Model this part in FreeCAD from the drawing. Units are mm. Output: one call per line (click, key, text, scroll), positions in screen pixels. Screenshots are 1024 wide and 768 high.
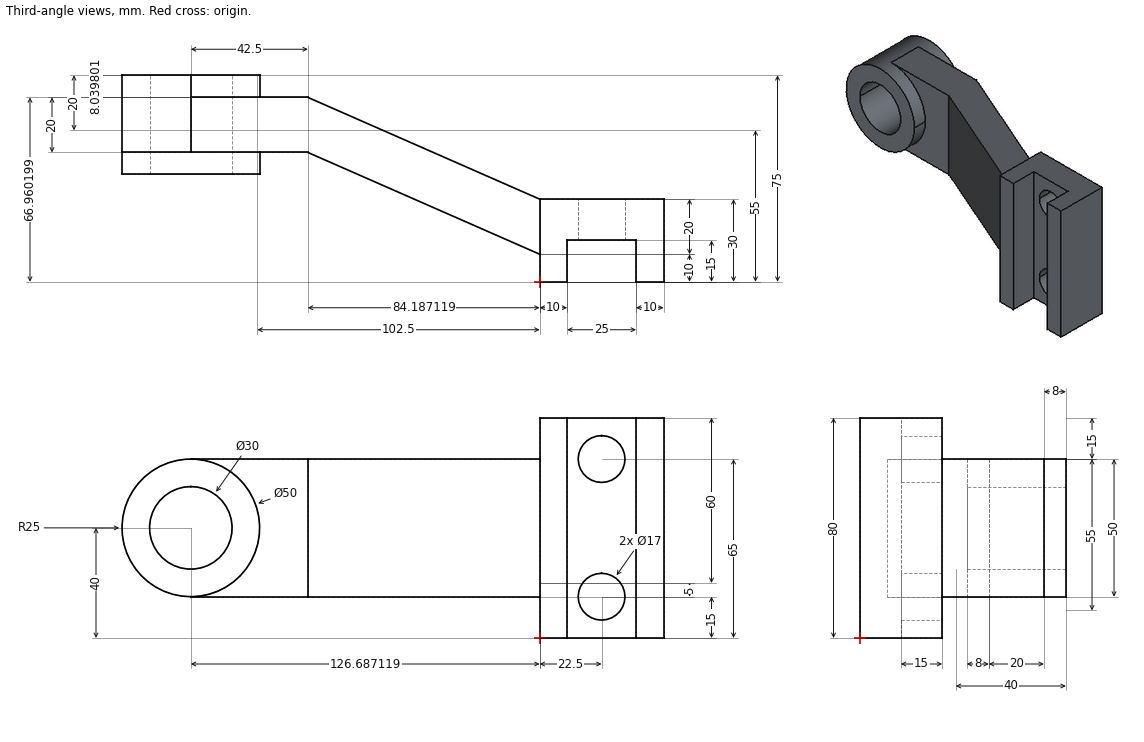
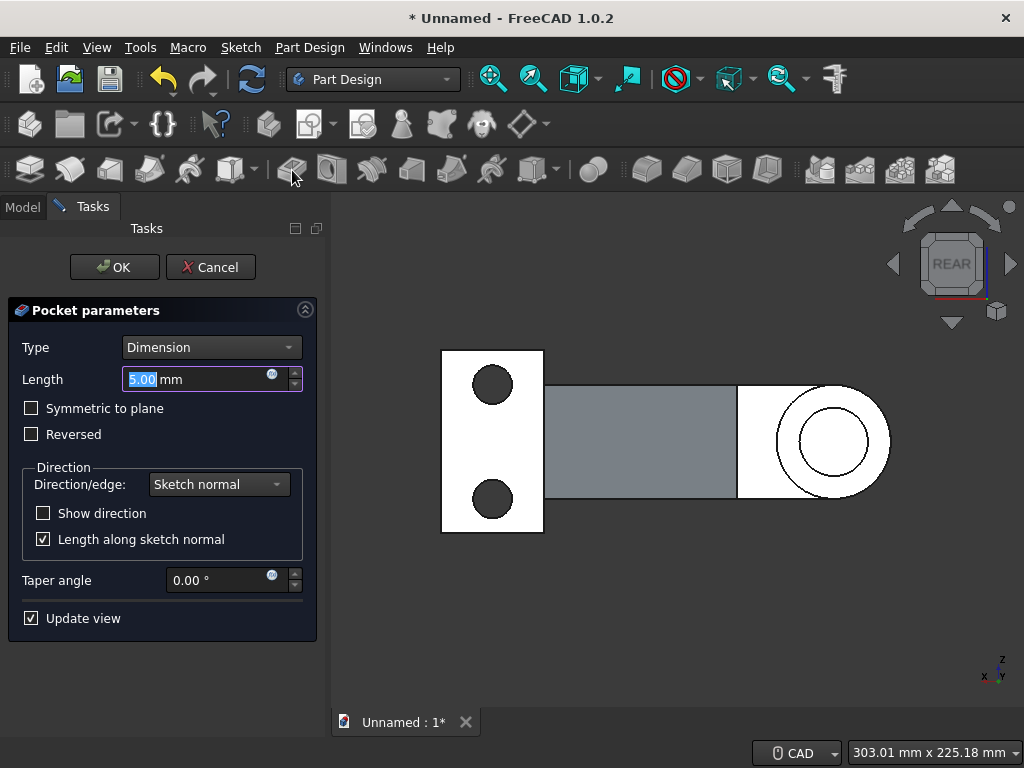
text(40)
key(Tab)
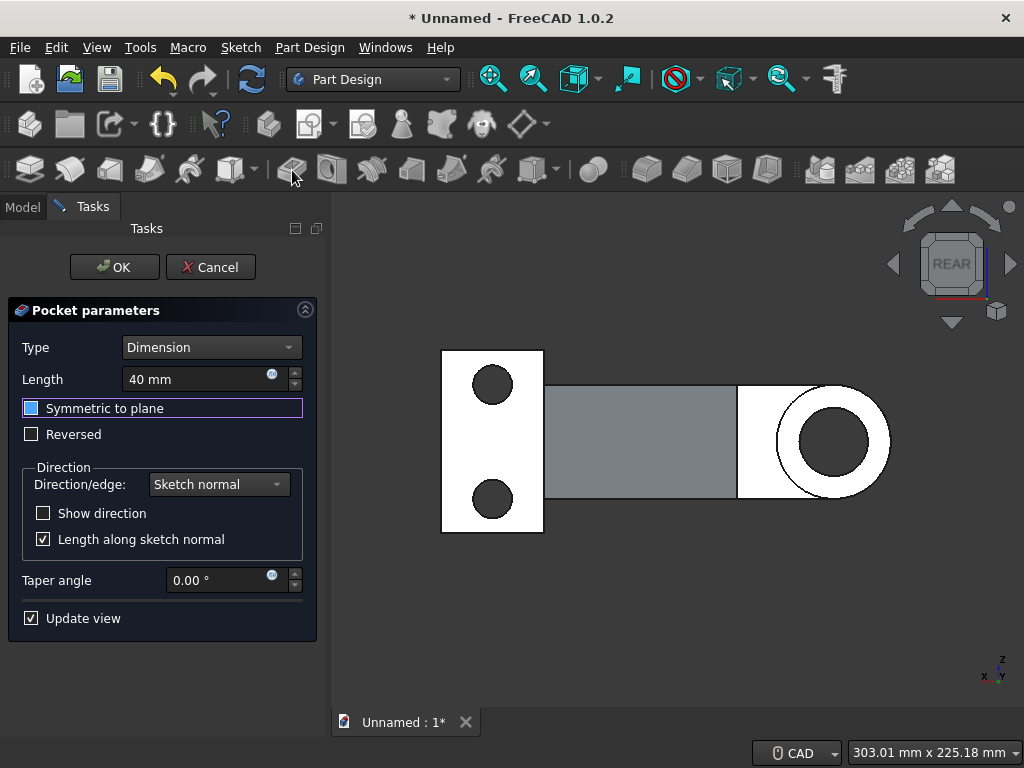
click(115, 267)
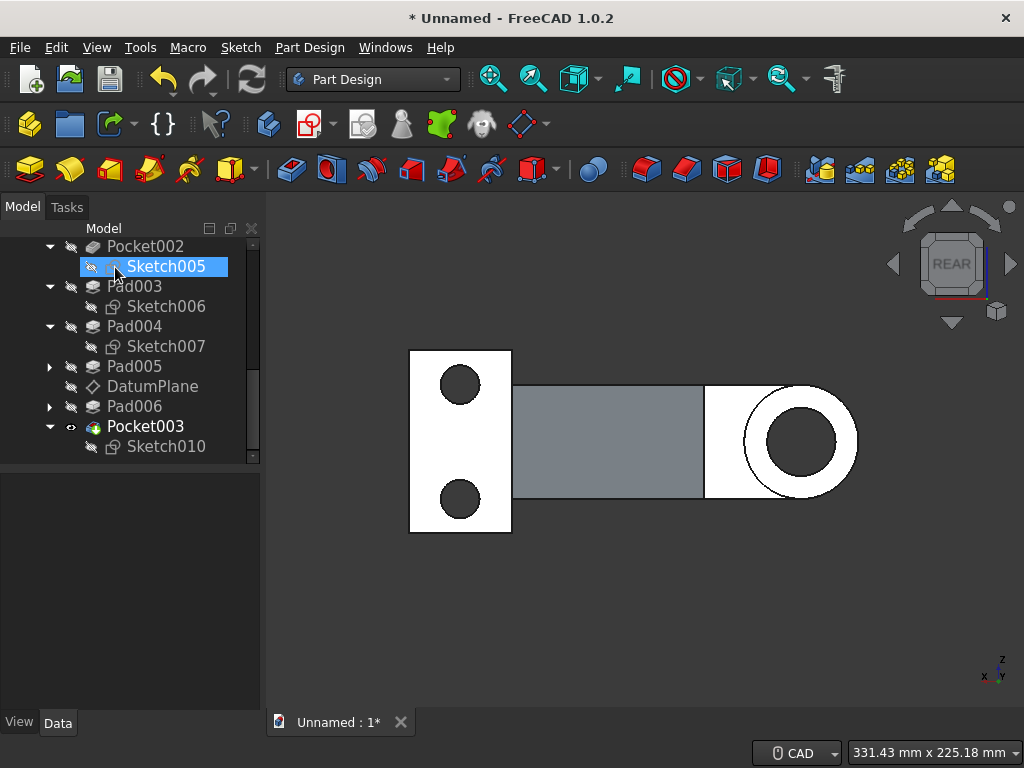
key(0)